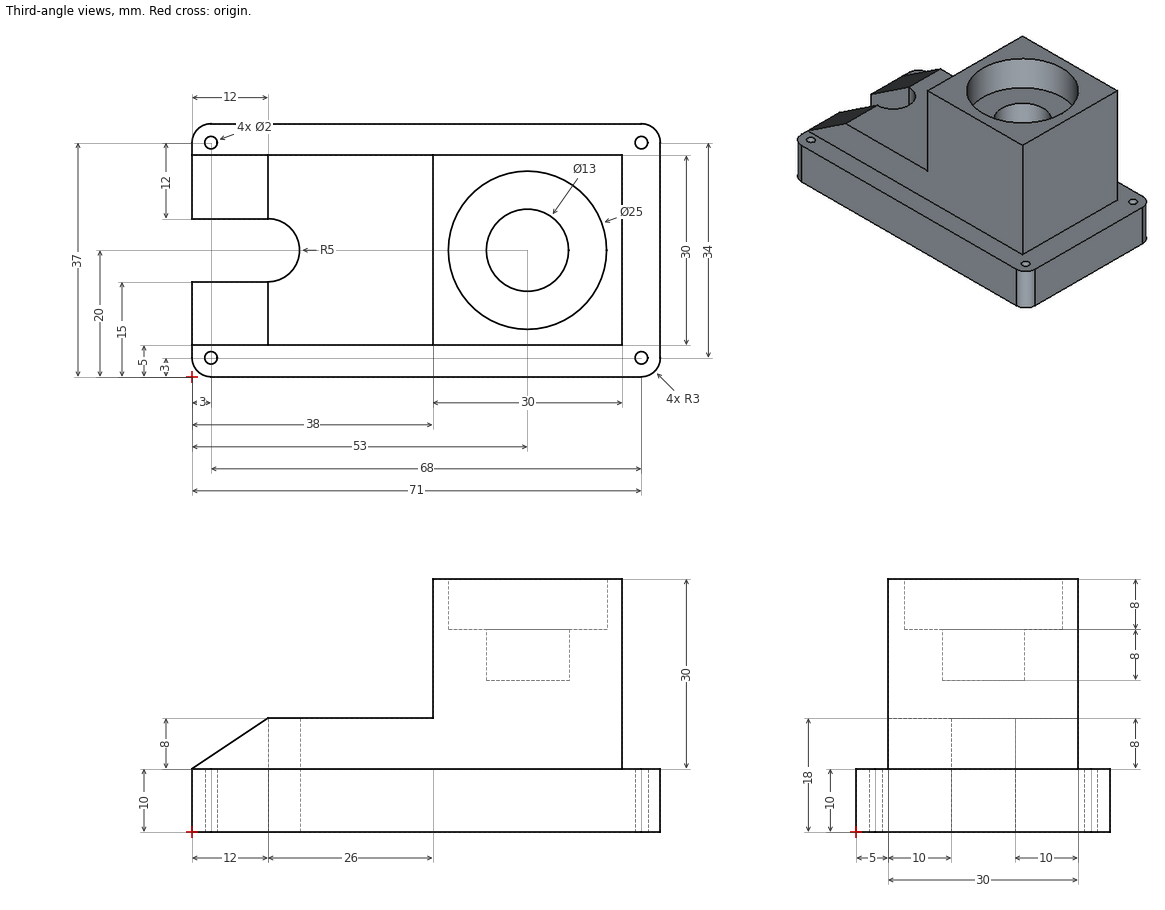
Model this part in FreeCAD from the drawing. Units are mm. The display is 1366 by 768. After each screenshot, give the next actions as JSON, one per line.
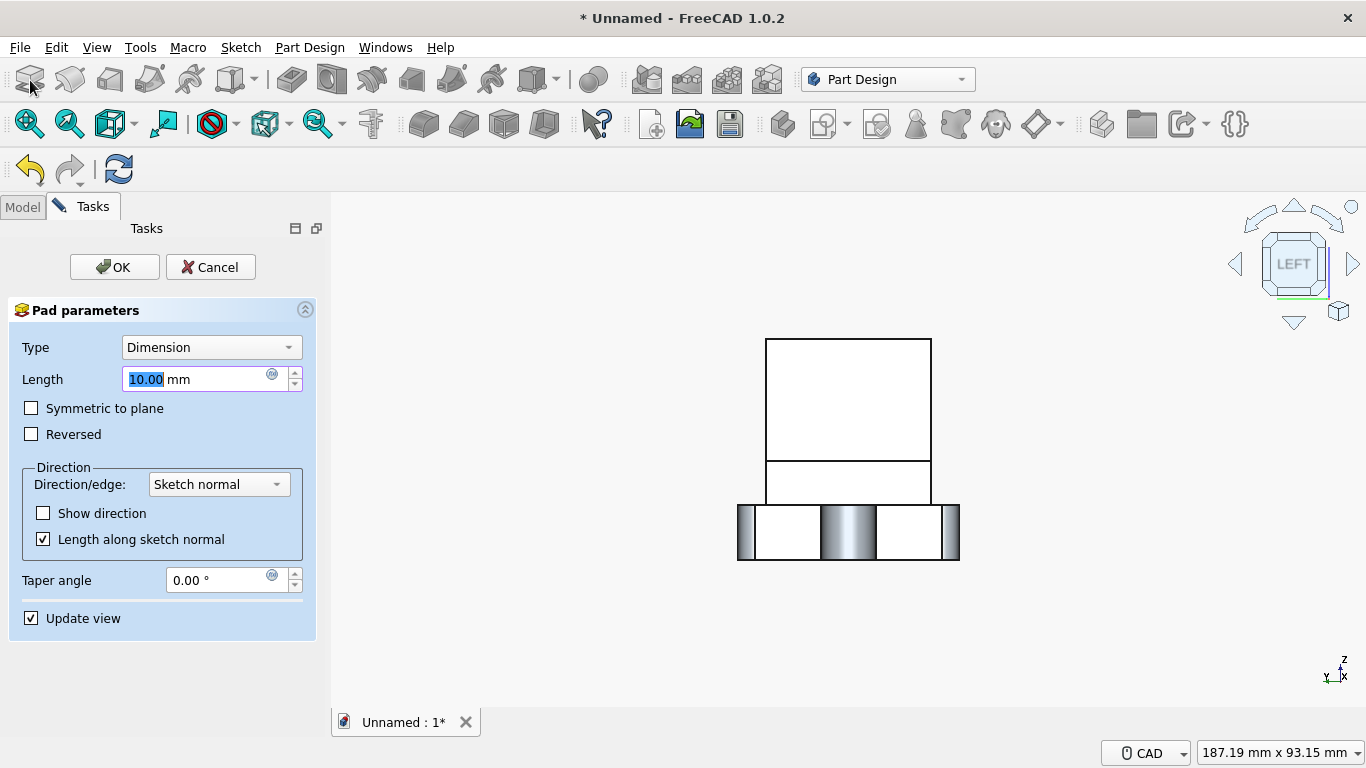
{"action": "type", "text": "26"}
{"action": "key", "text": "Tab"}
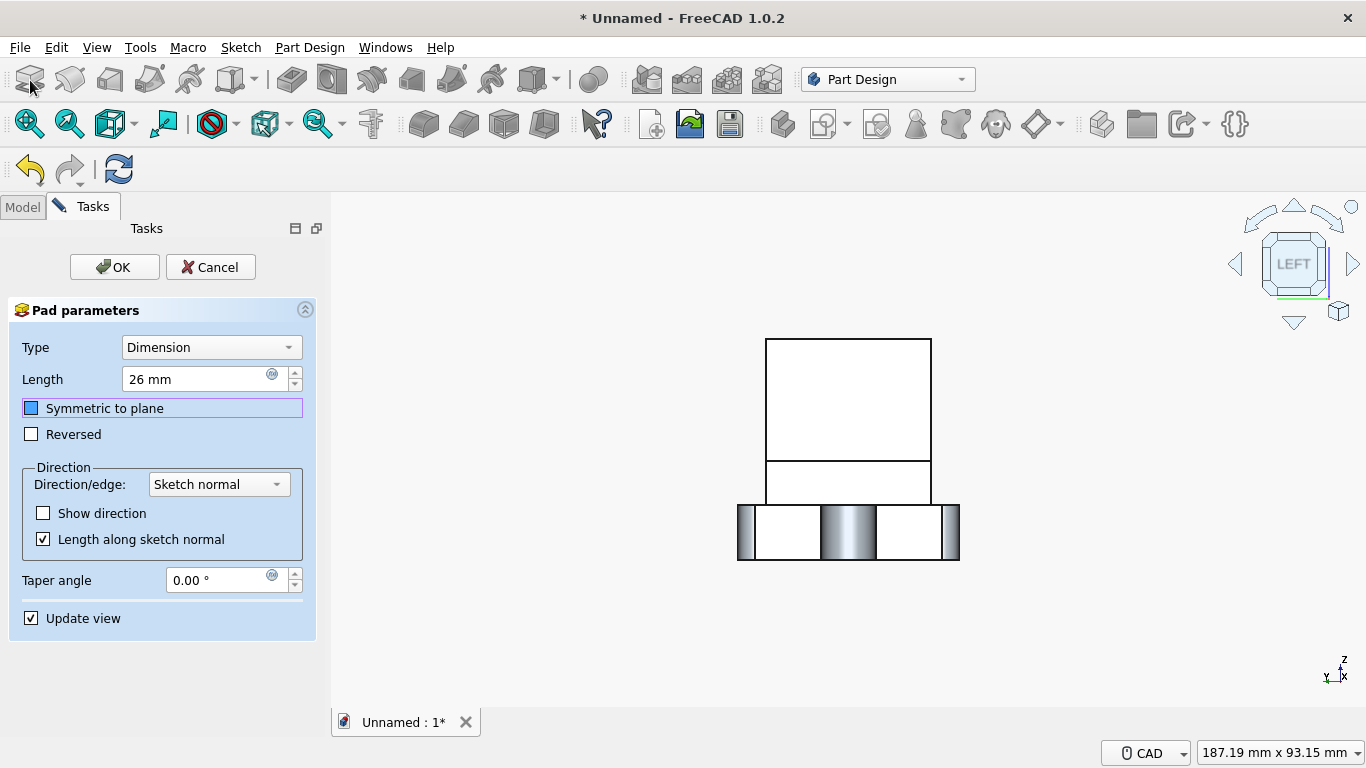
{"action": "left_click", "coordinate": [115, 267]}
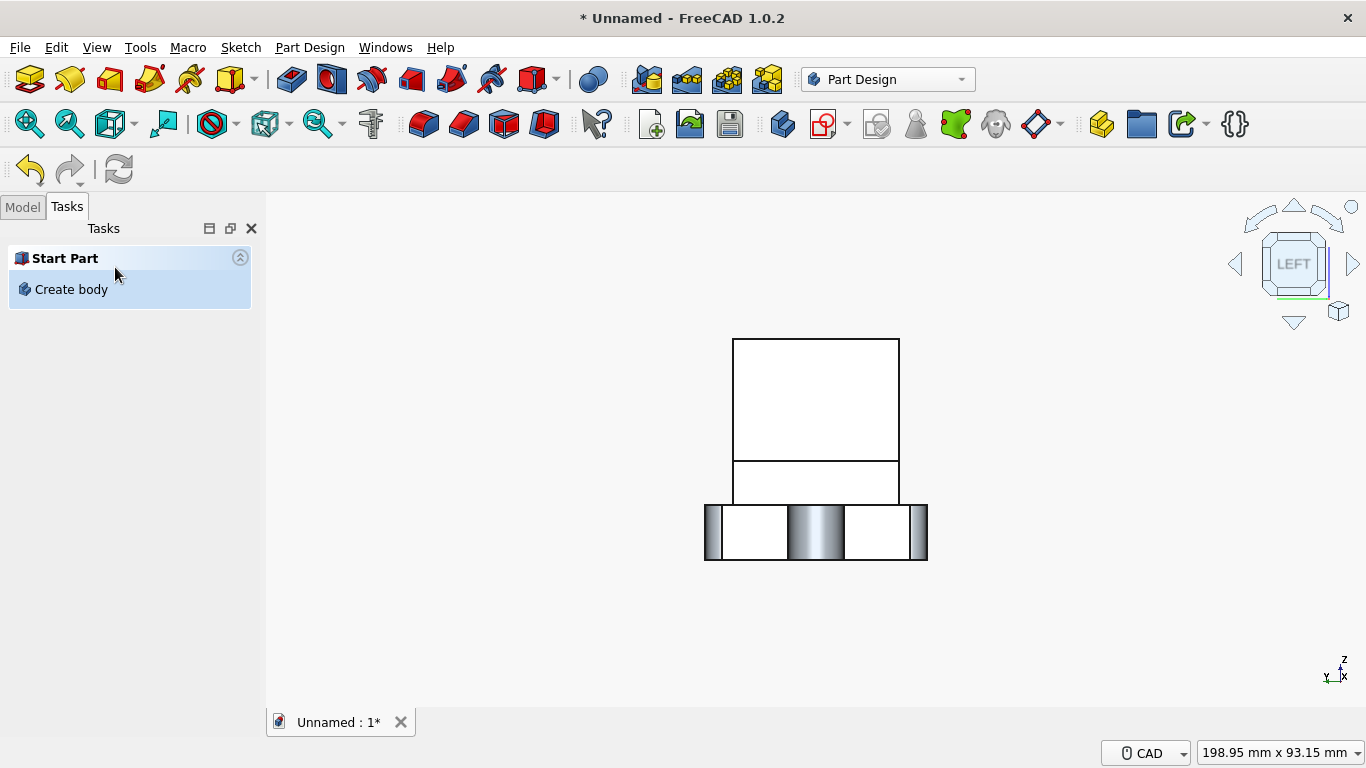
{"action": "left_click", "coordinate": [30, 124]}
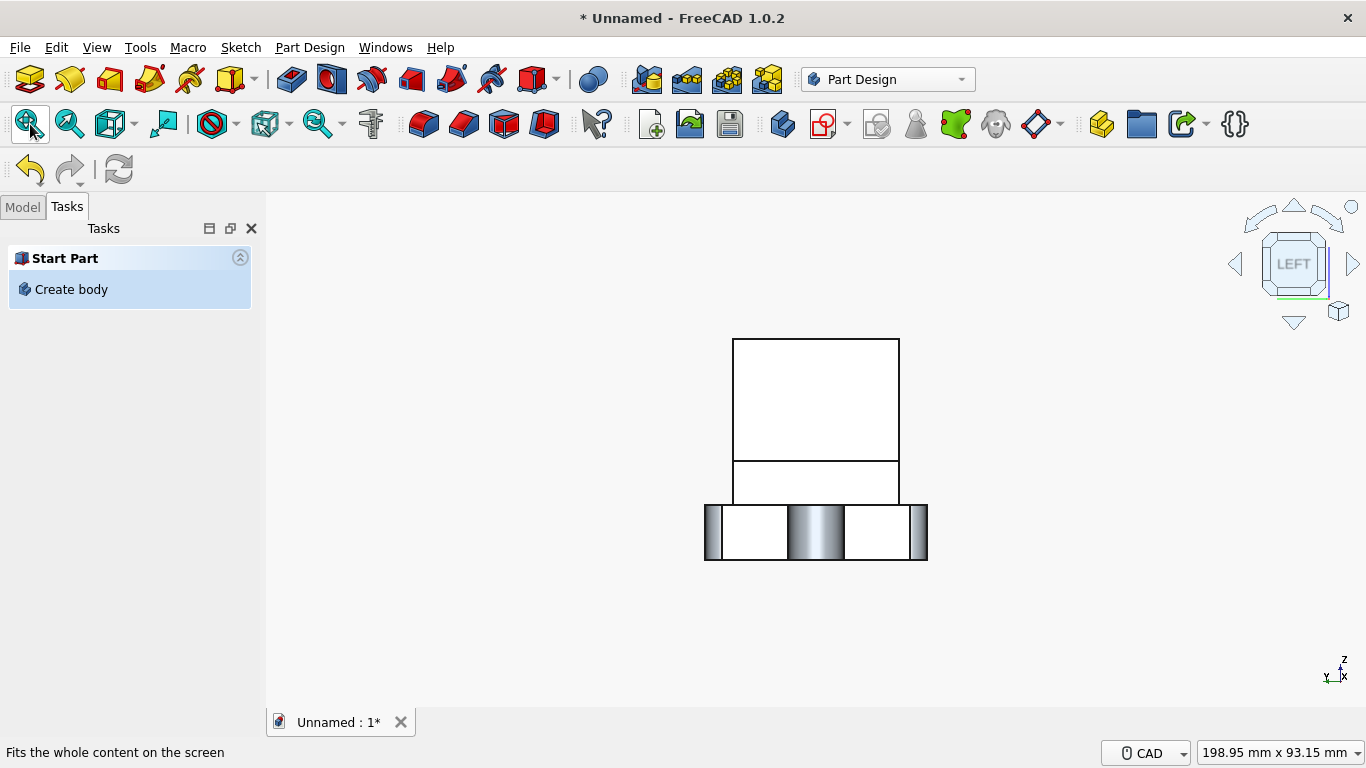
{"action": "key", "text": "0"}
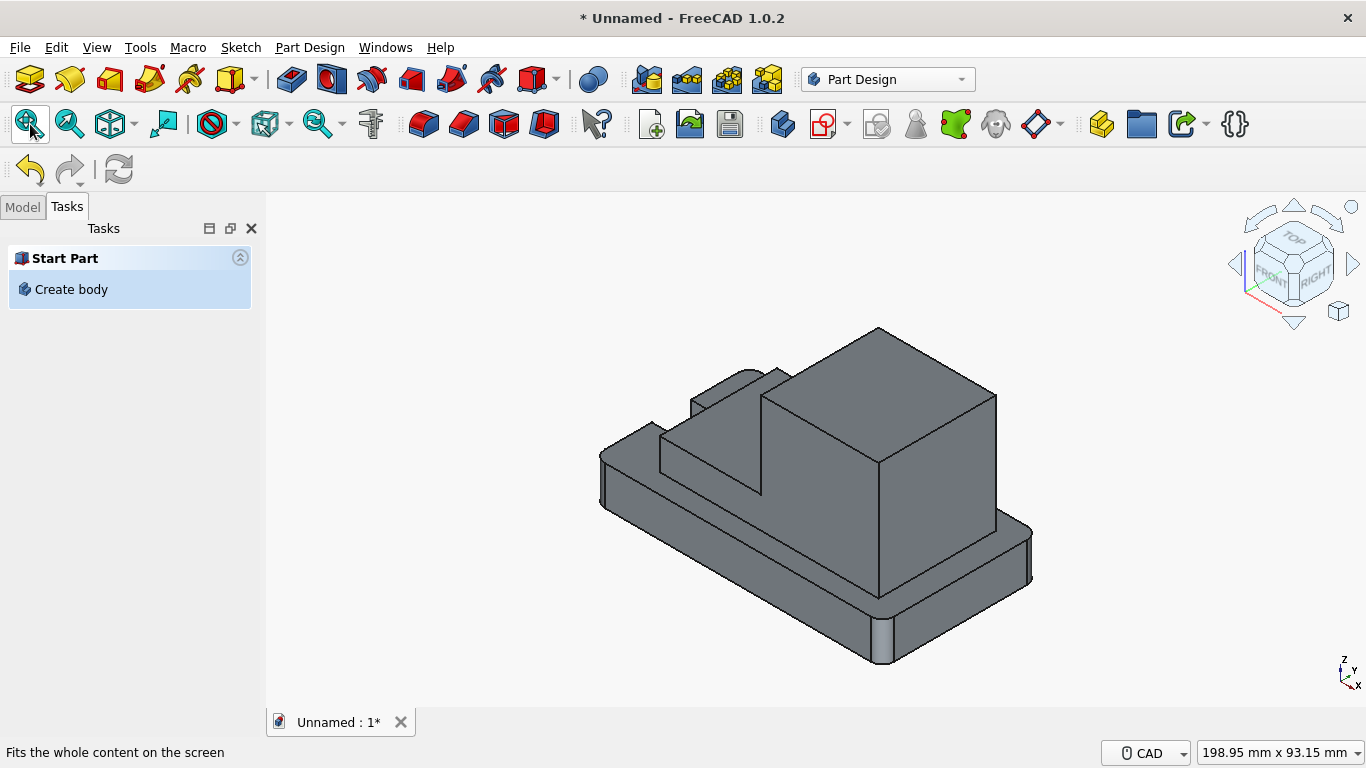
{"action": "left_click", "coordinate": [647, 448]}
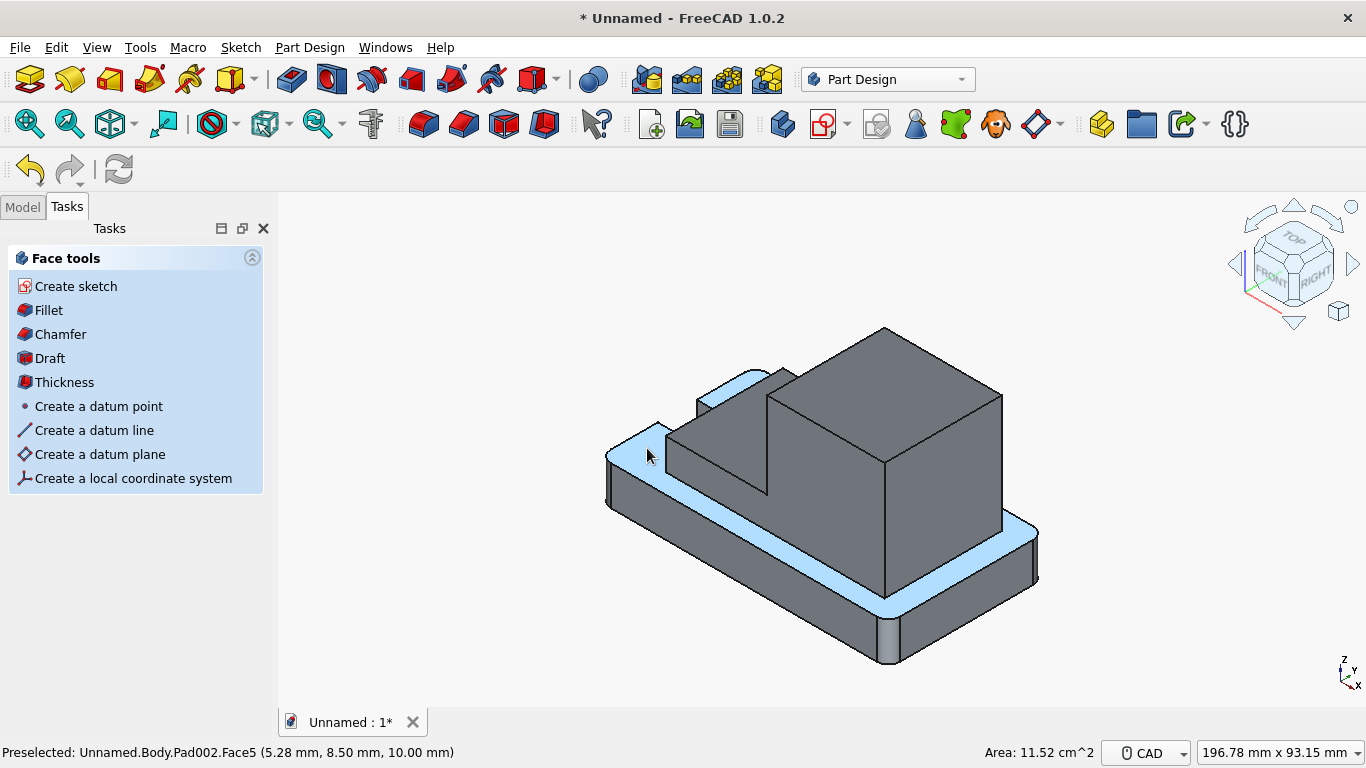
{"action": "left_click", "coordinate": [824, 124]}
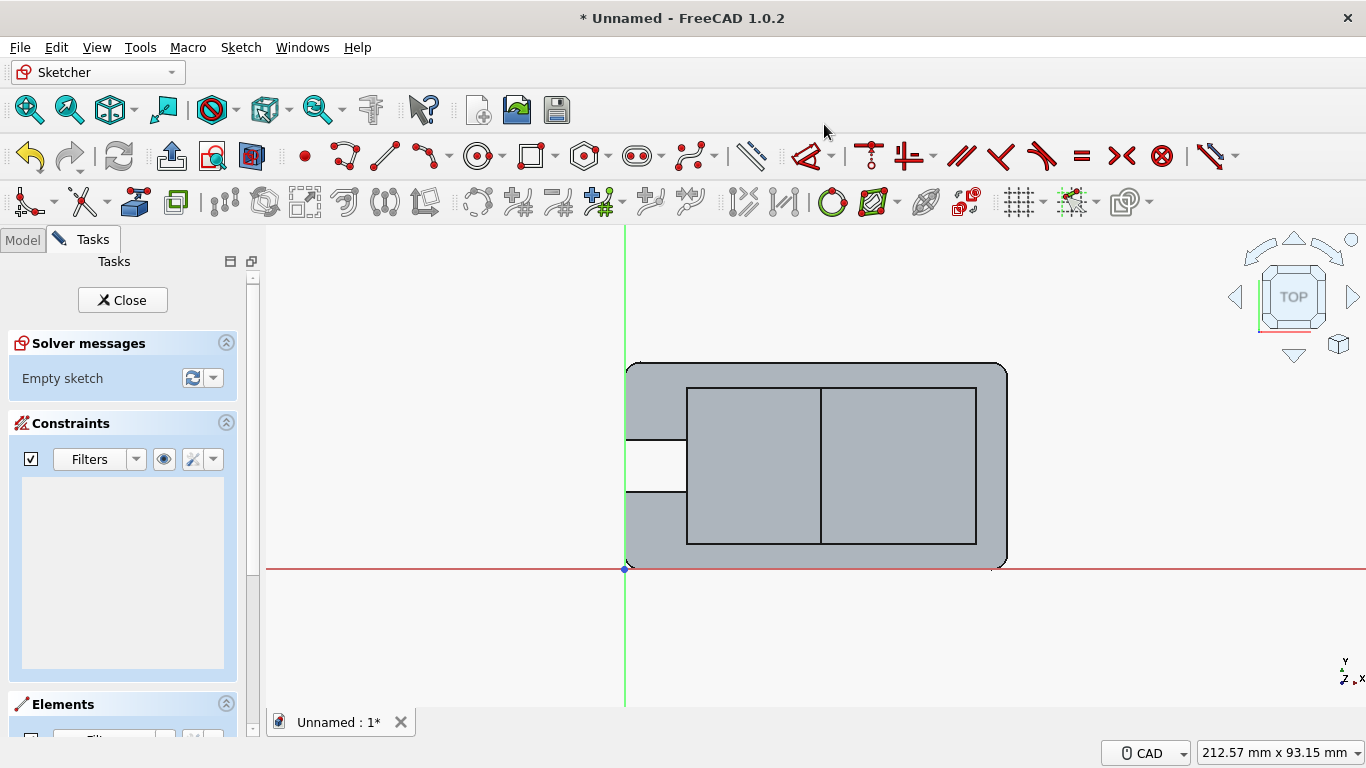
{"action": "scroll", "coordinate": [690, 466], "scroll_direction": "up", "scroll_amount": 9}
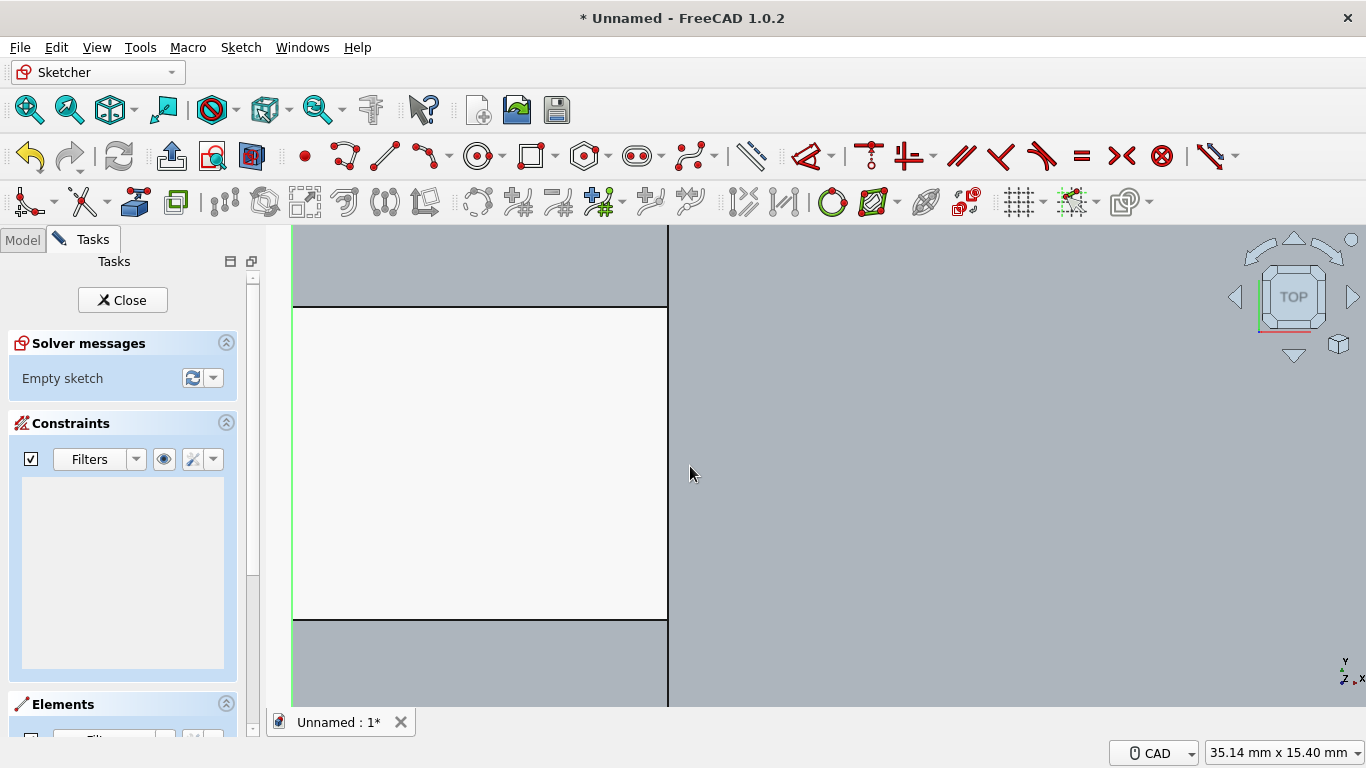
{"action": "left_click", "coordinate": [386, 156]}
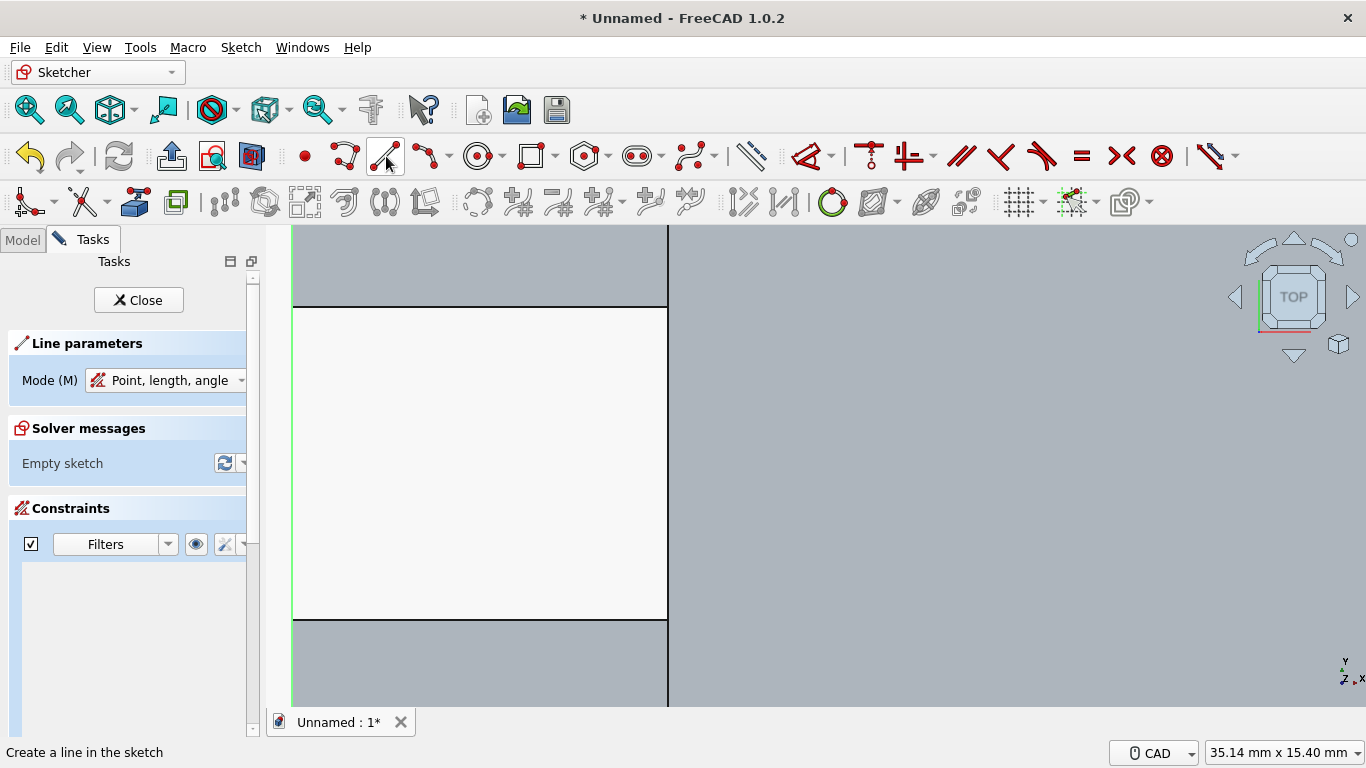
{"action": "left_click", "coordinate": [668, 620]}
{"action": "left_click", "coordinate": [668, 307]}